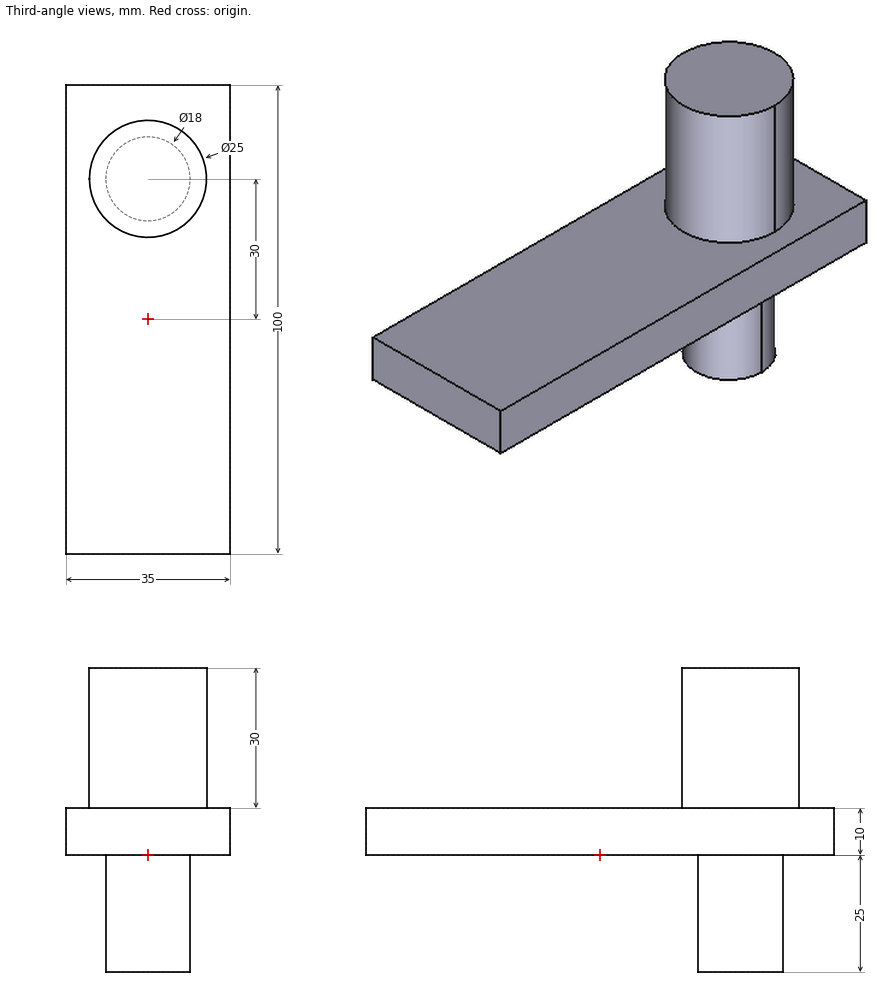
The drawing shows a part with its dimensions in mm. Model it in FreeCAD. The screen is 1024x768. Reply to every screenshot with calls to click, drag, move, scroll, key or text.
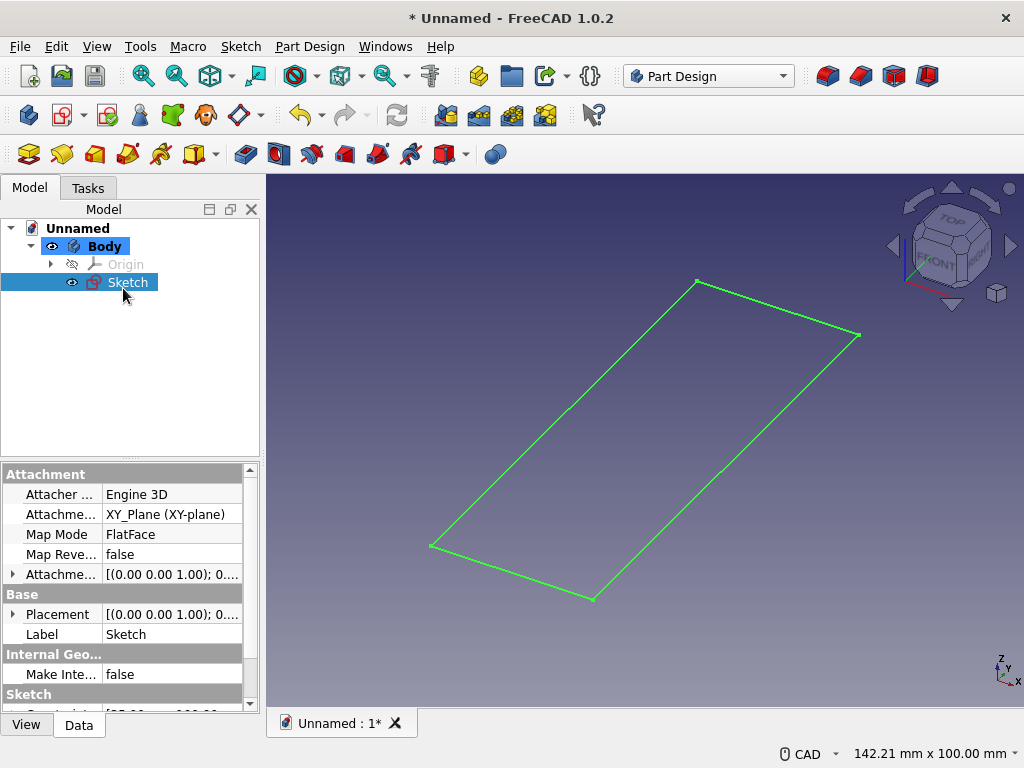
click(29, 154)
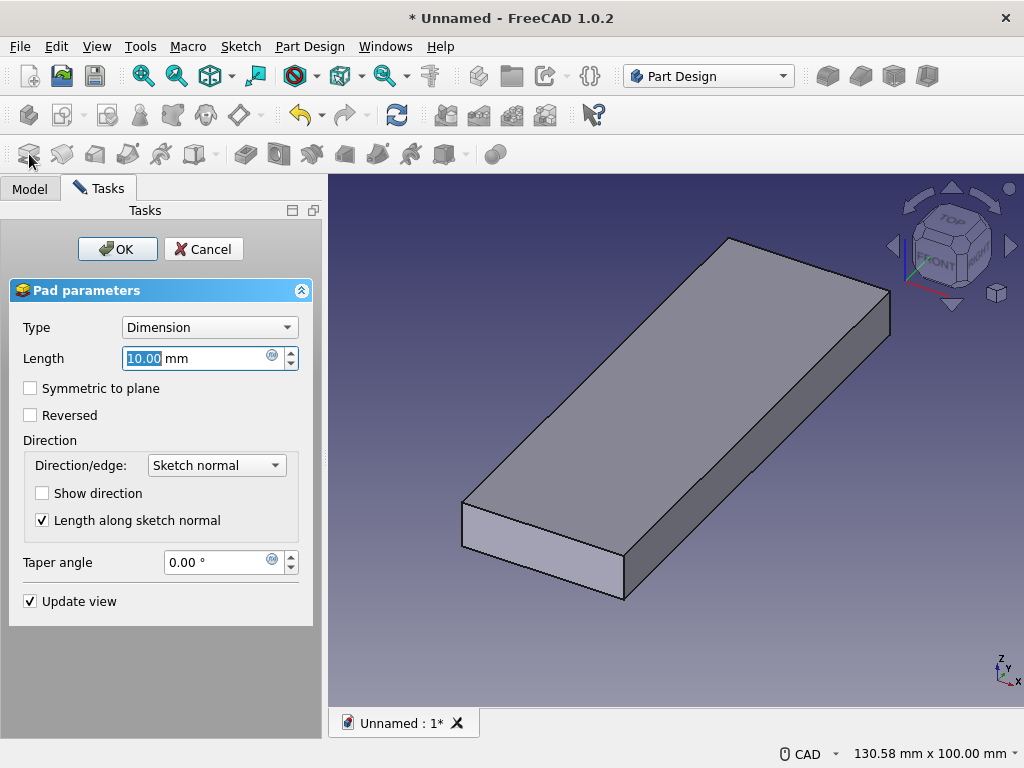
text(10)
key(Tab)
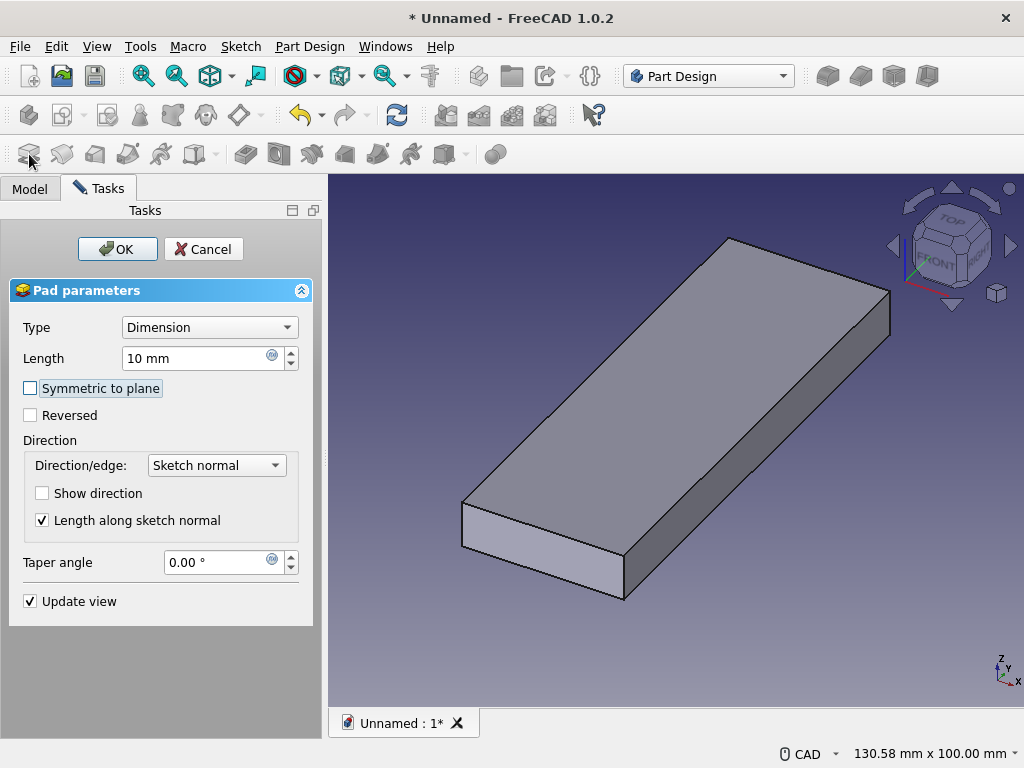
click(118, 249)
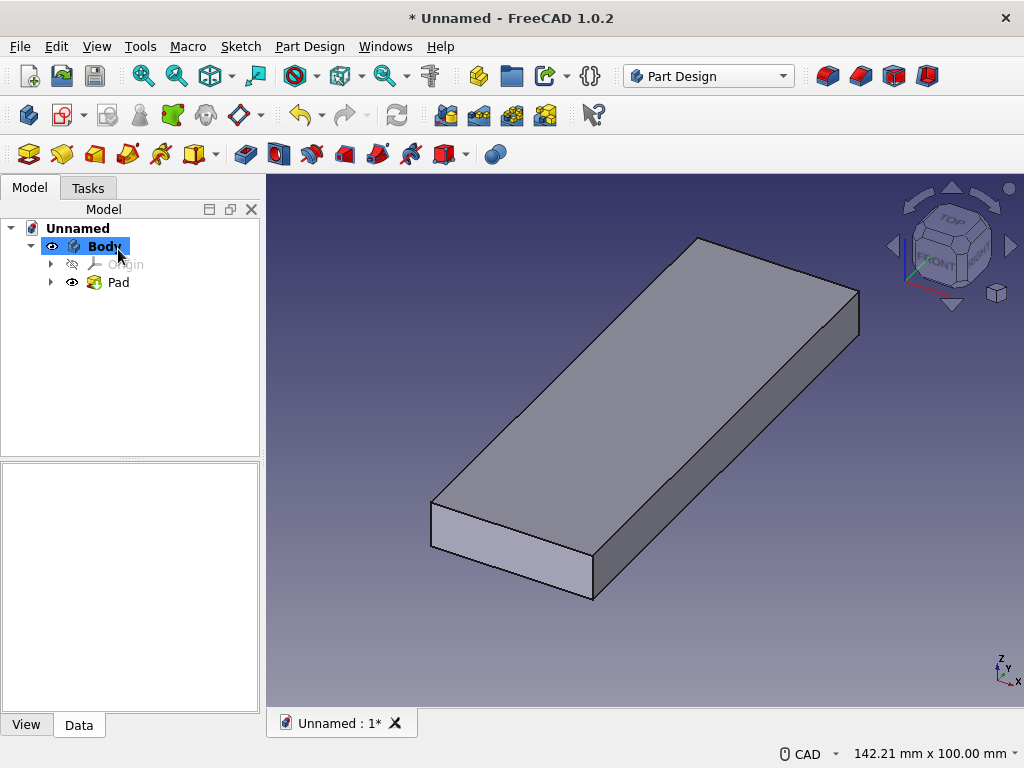
click(721, 320)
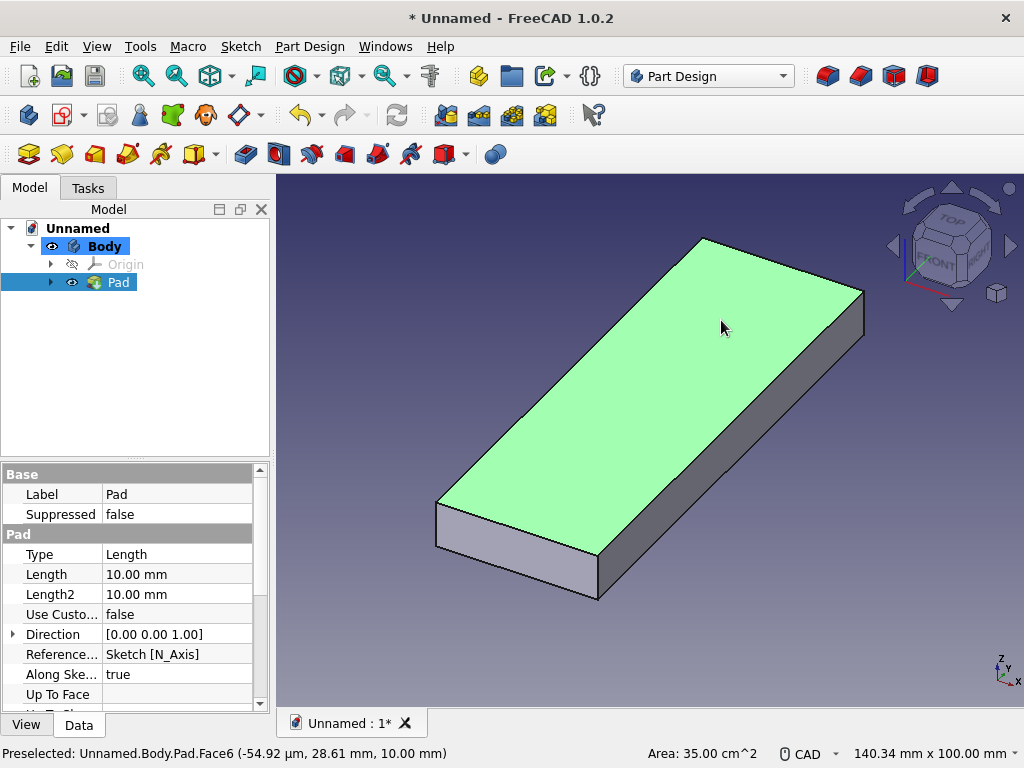
click(62, 116)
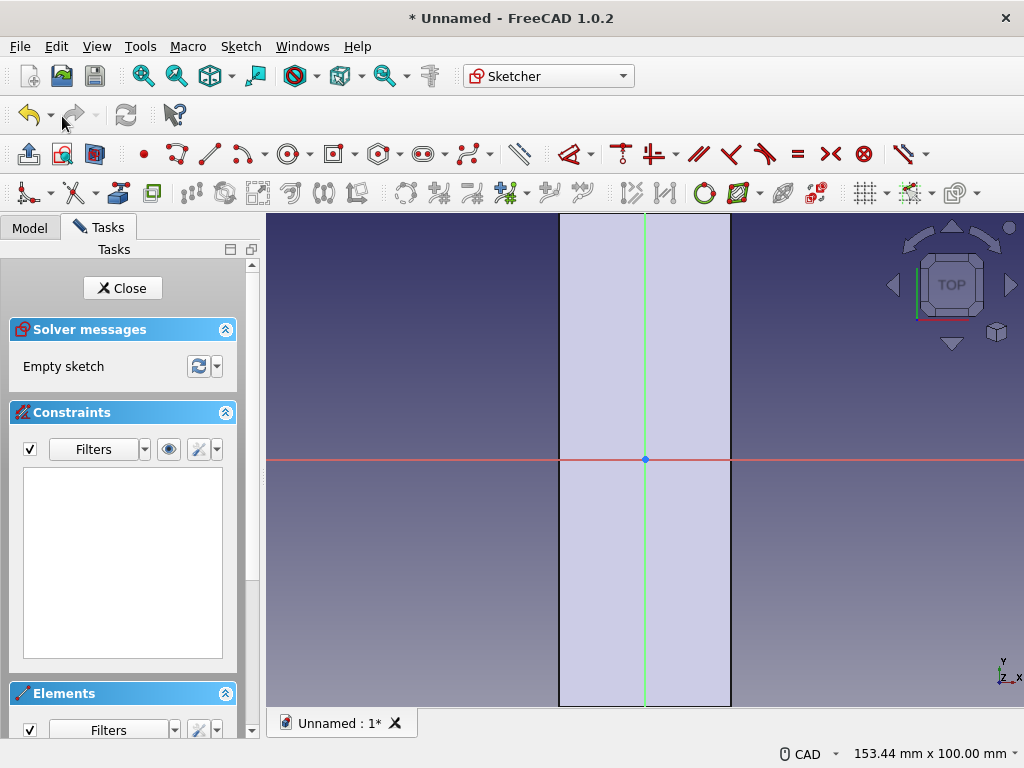
scroll(294, 679, down, 1)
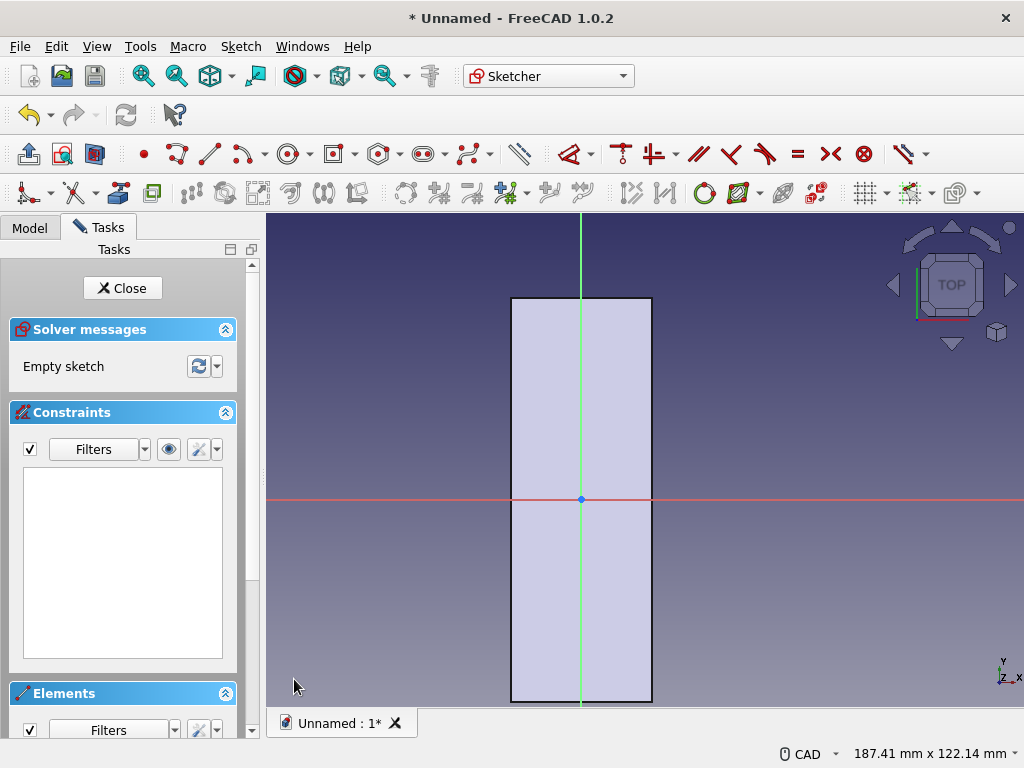
scroll(587, 358, up, 3)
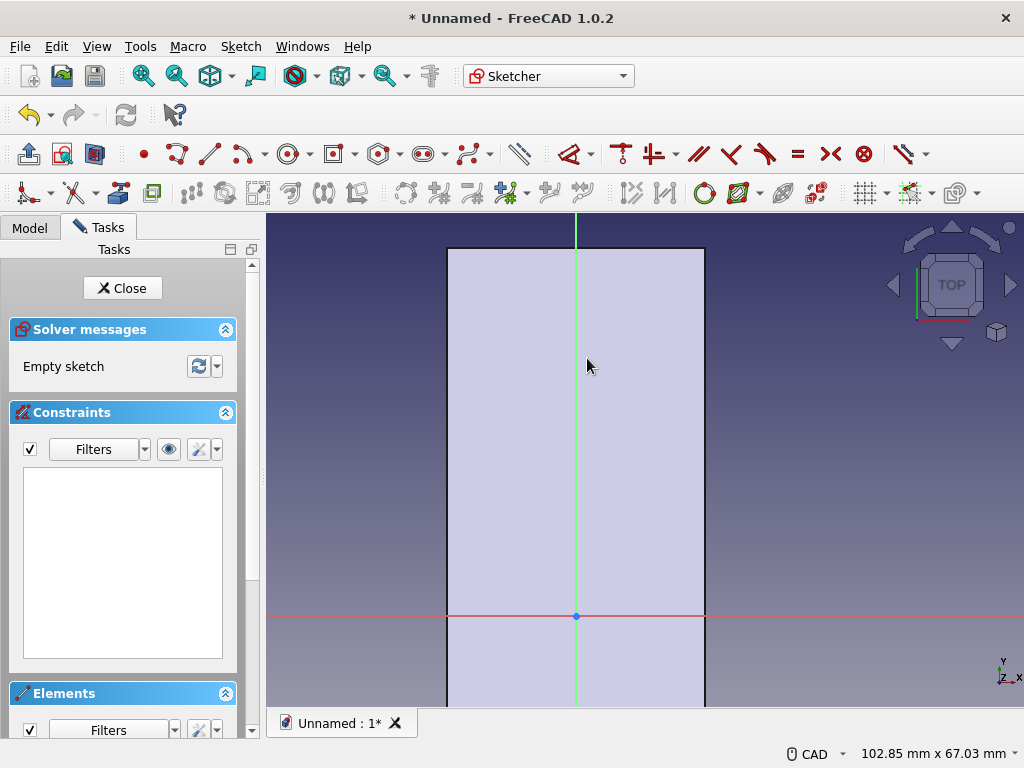
click(288, 154)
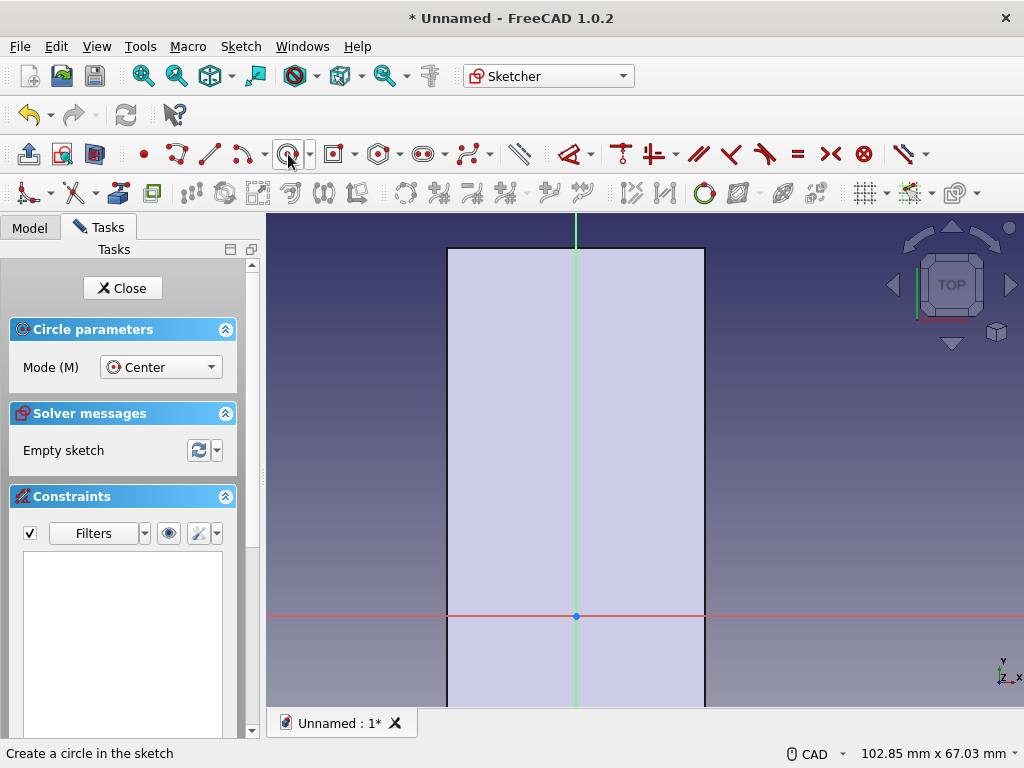
click(576, 395)
click(642, 330)
key(Escape)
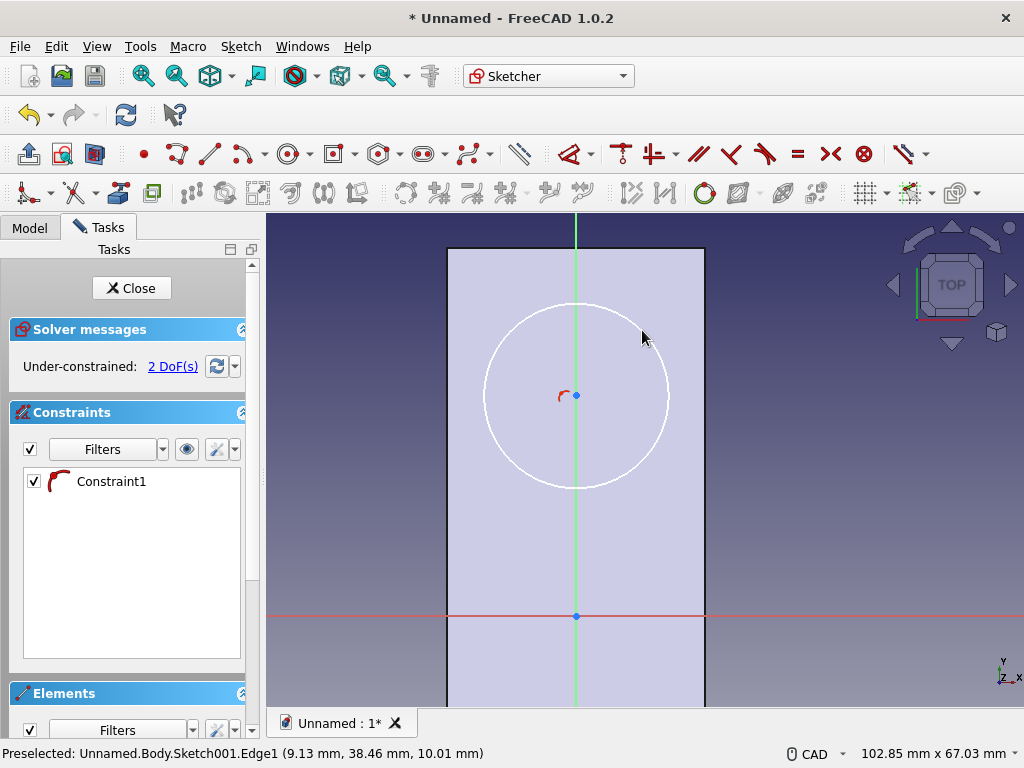
click(568, 154)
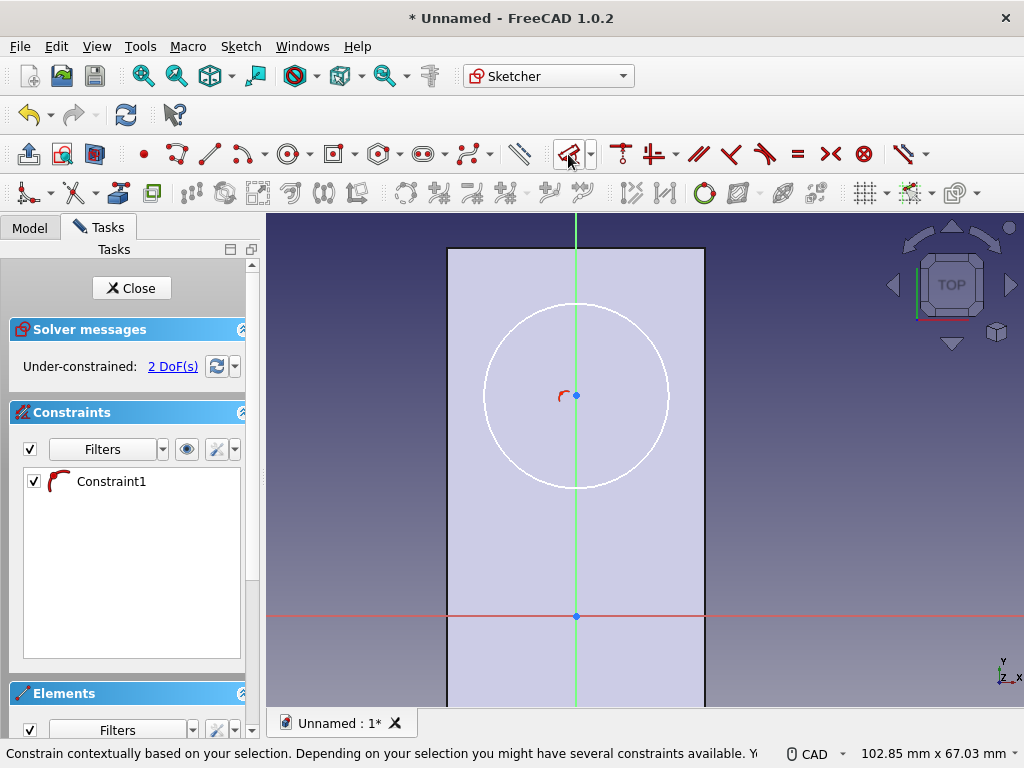
click(642, 331)
click(665, 308)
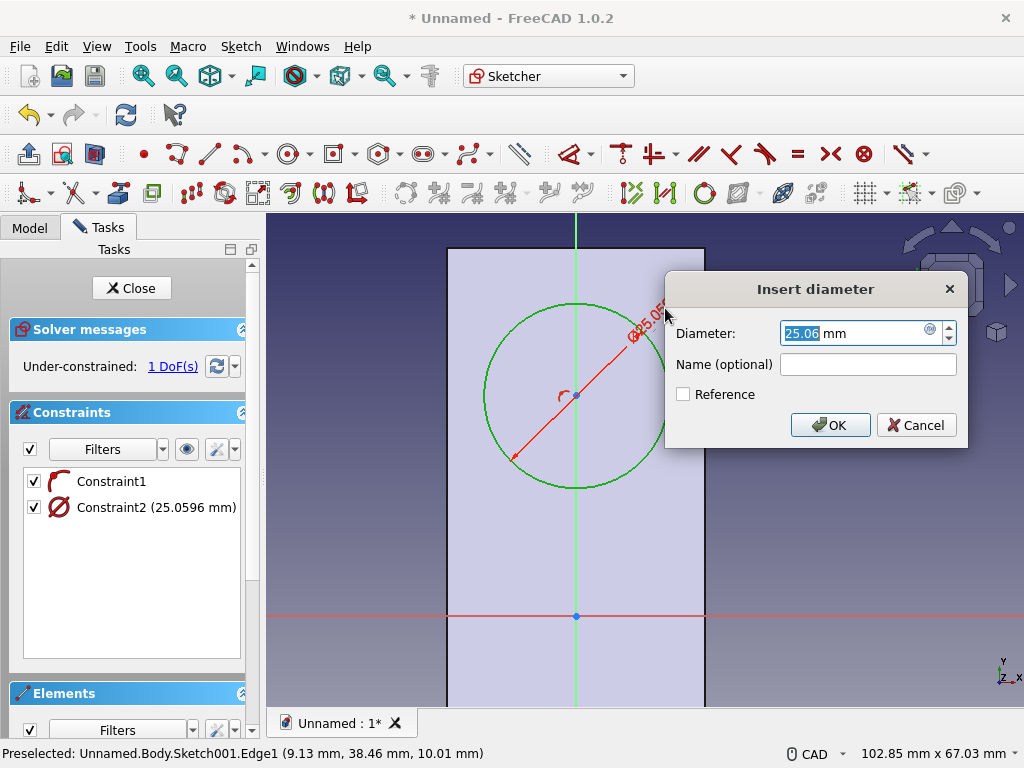
text(25)
key(Return)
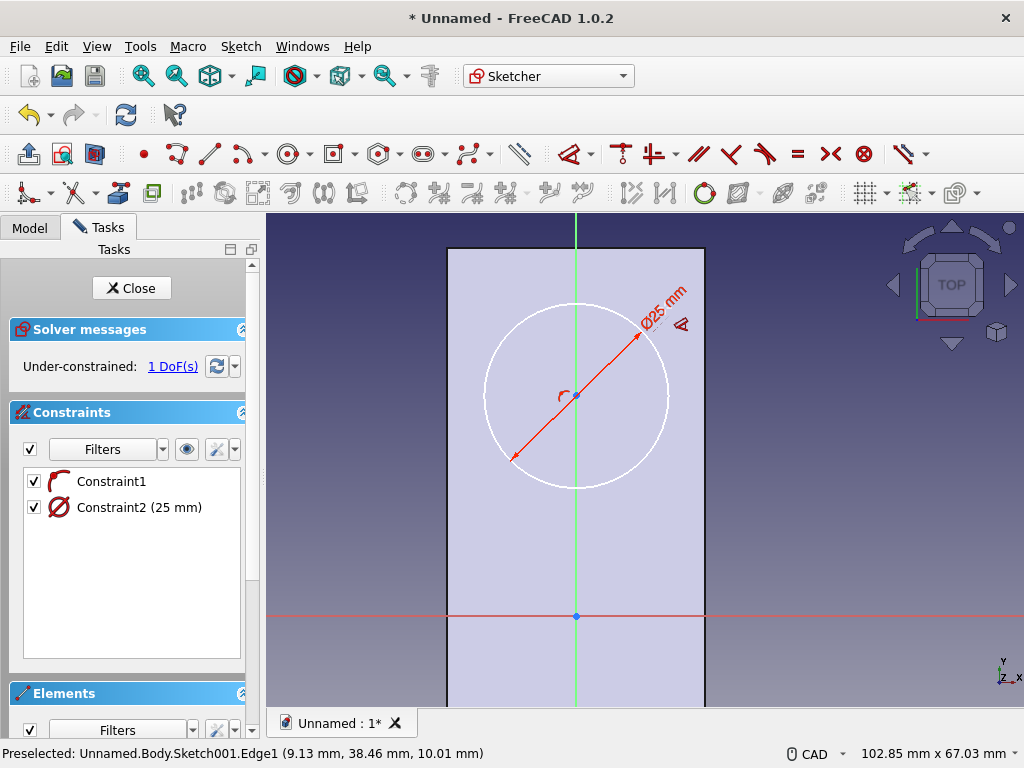
click(576, 396)
click(610, 506)